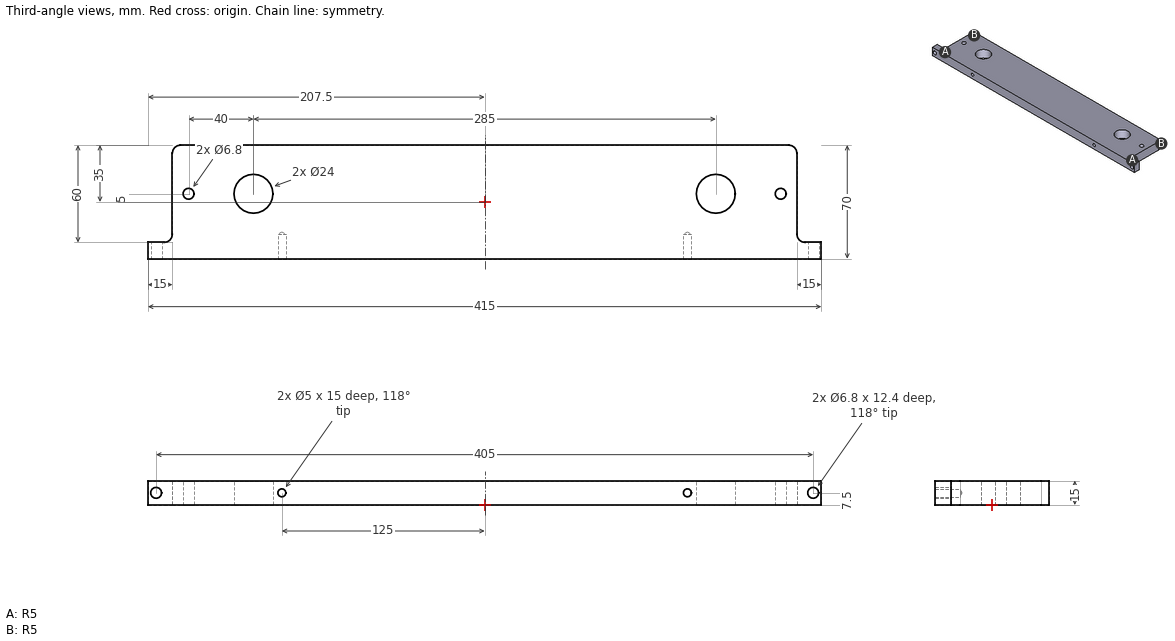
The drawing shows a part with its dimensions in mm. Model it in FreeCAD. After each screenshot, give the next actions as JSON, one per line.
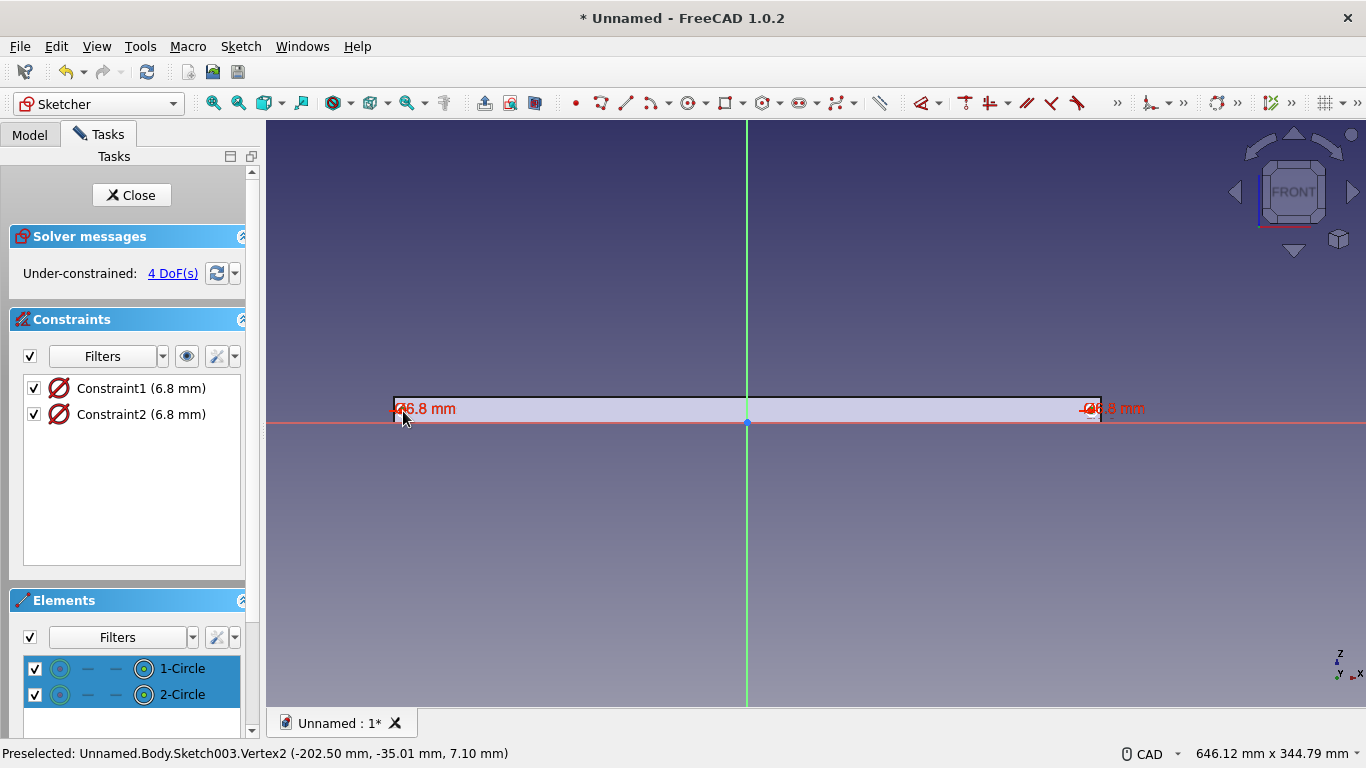
{"action": "left_click", "coordinate": [747, 641]}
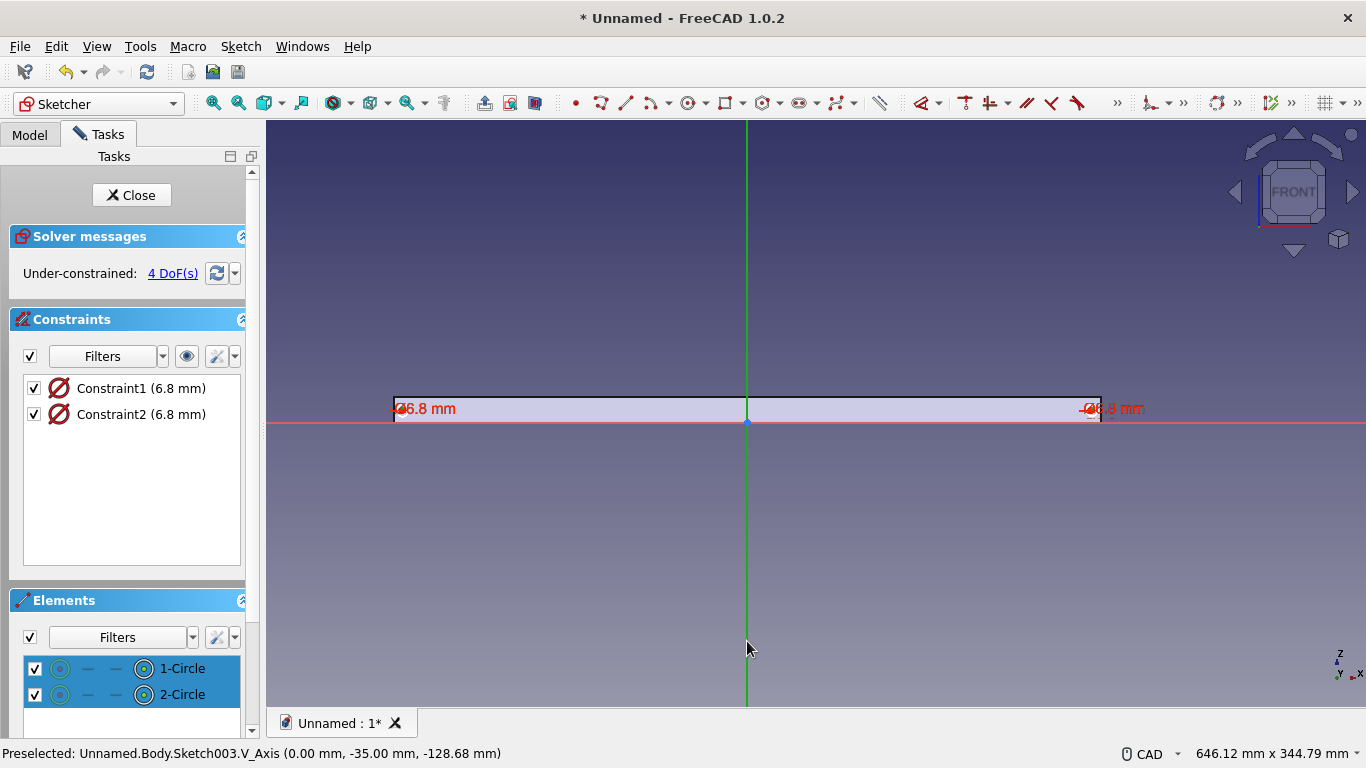
{"action": "key", "text": "s"}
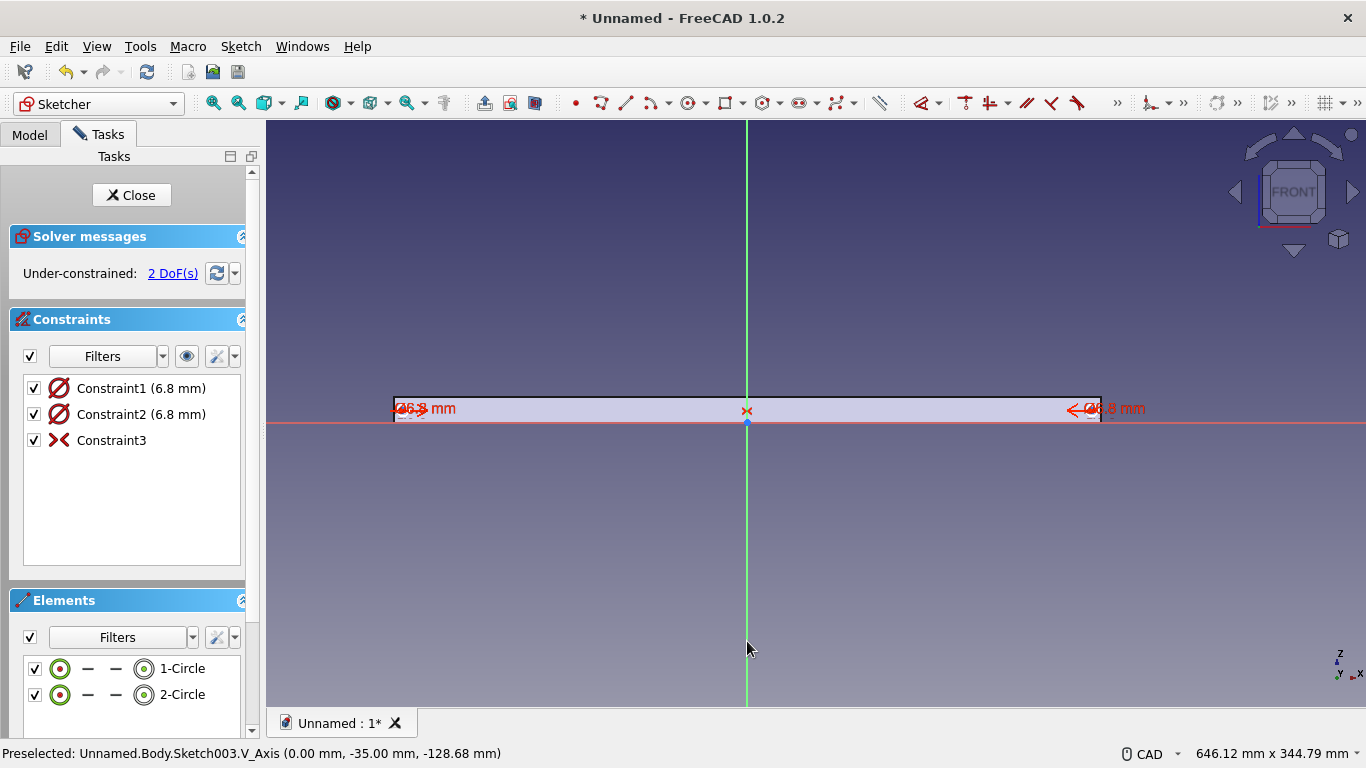
{"action": "key", "text": "d"}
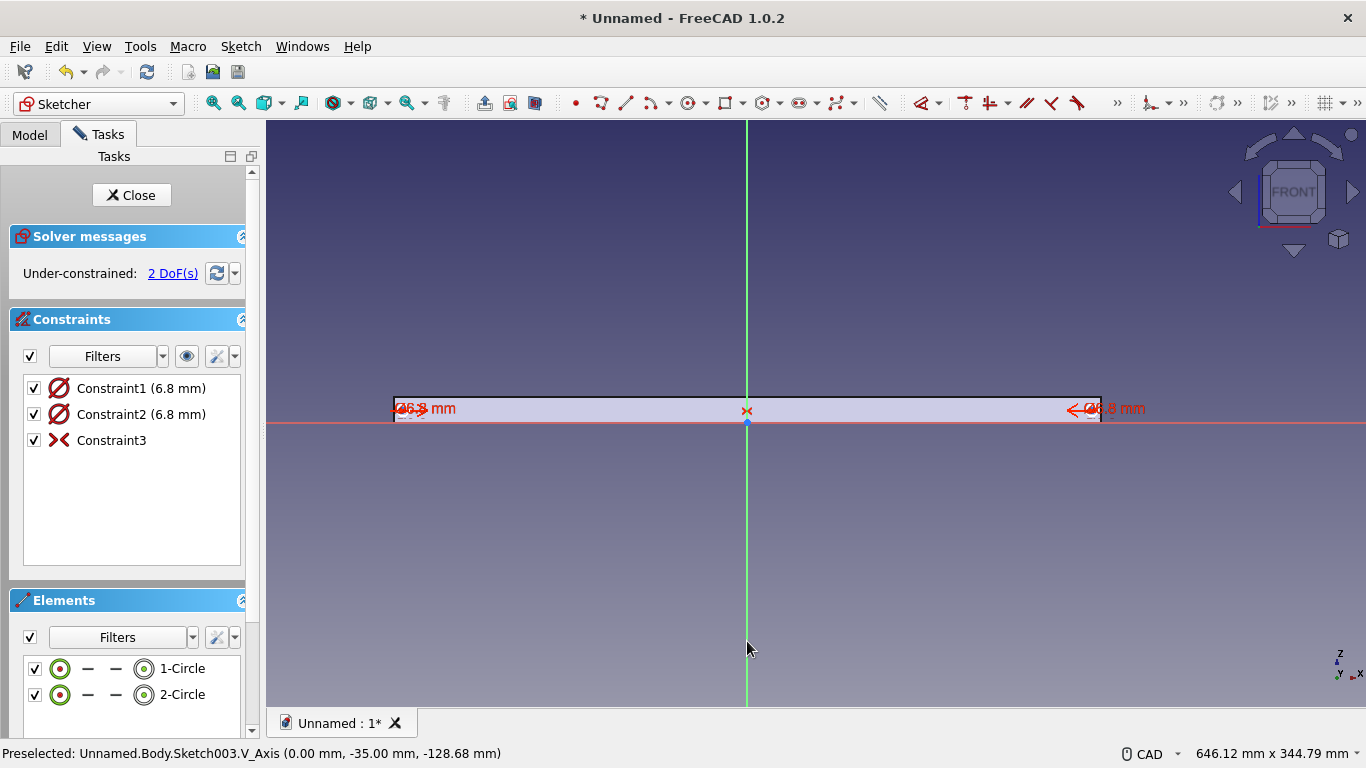
{"action": "scroll", "coordinate": [1092, 411], "scroll_direction": "up", "scroll_amount": 6}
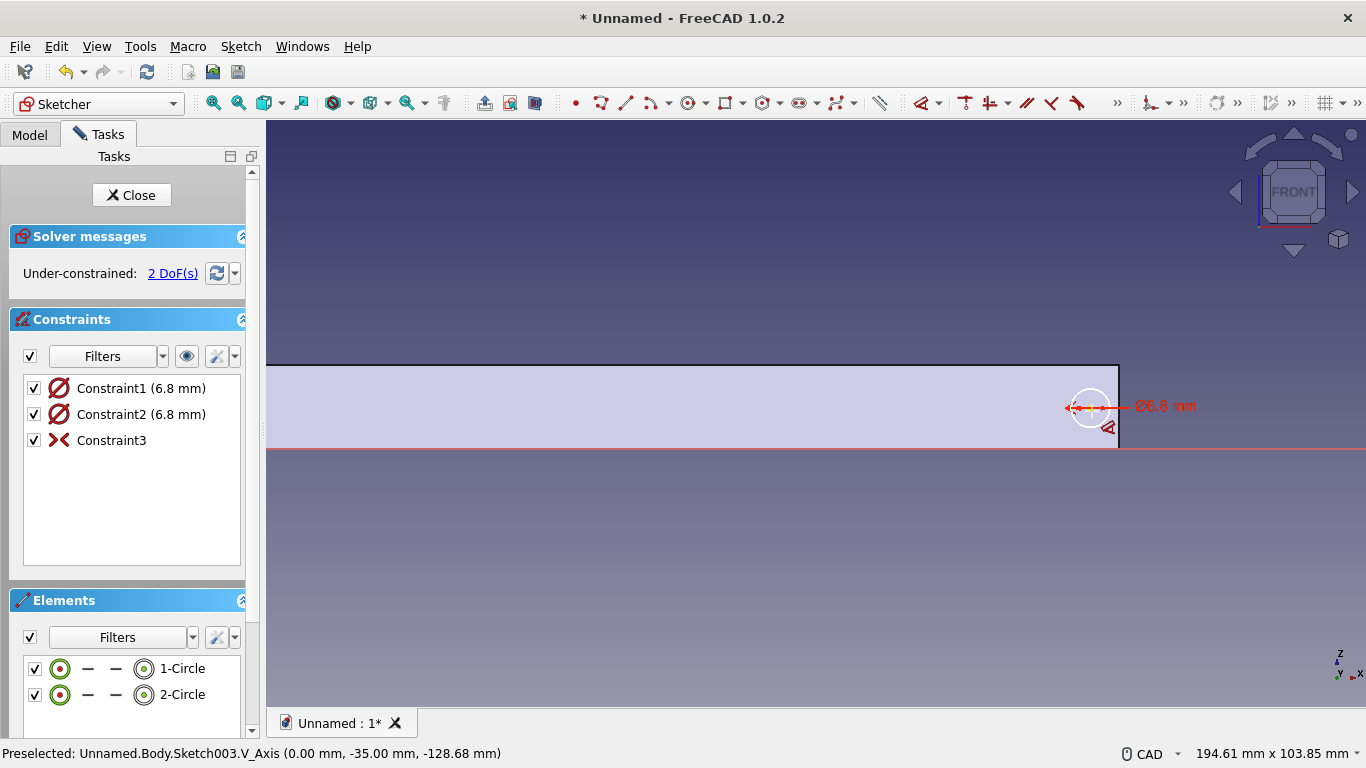
{"action": "left_click", "coordinate": [1091, 408]}
{"action": "left_click", "coordinate": [1125, 429]}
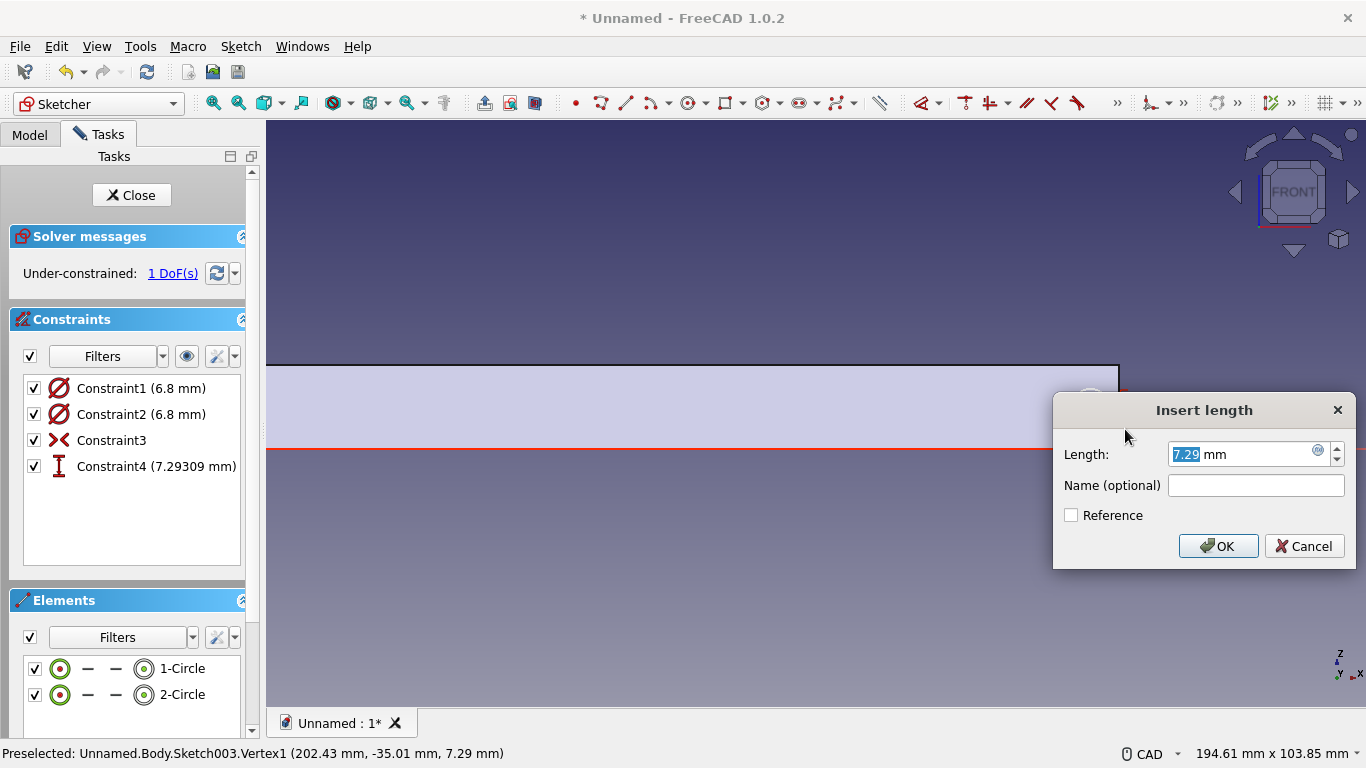
{"action": "type", "text": "7.5"}
{"action": "key", "text": "Return"}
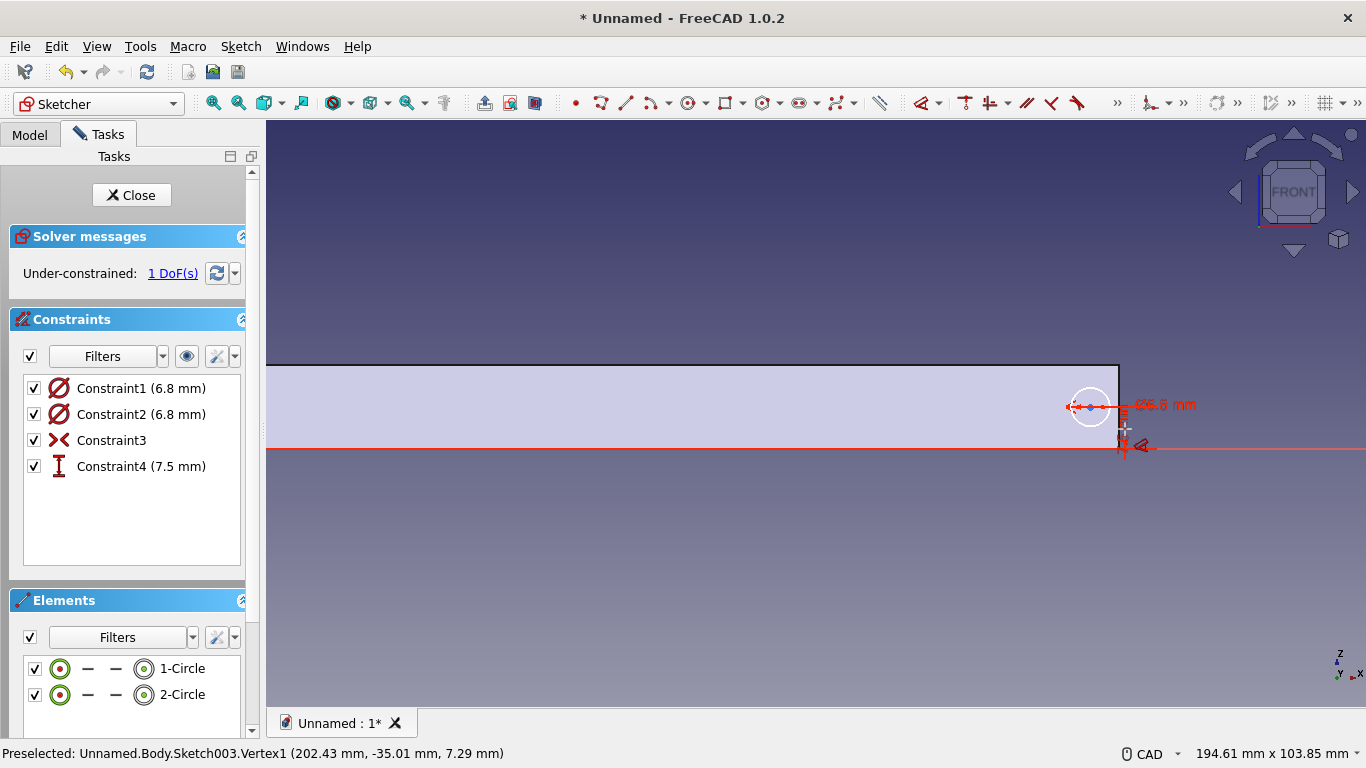
{"action": "scroll", "coordinate": [1093, 411], "scroll_direction": "down", "scroll_amount": 6}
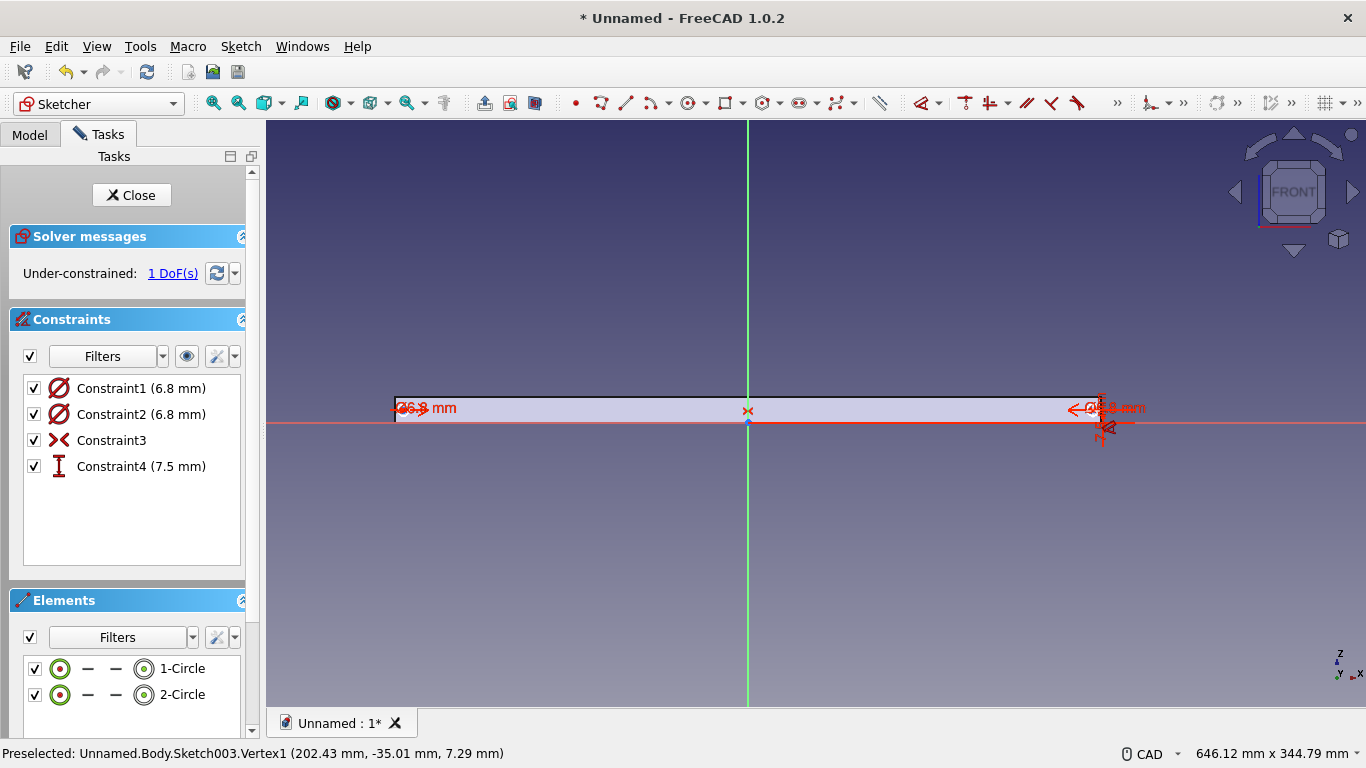
{"action": "left_click", "coordinate": [1093, 410]}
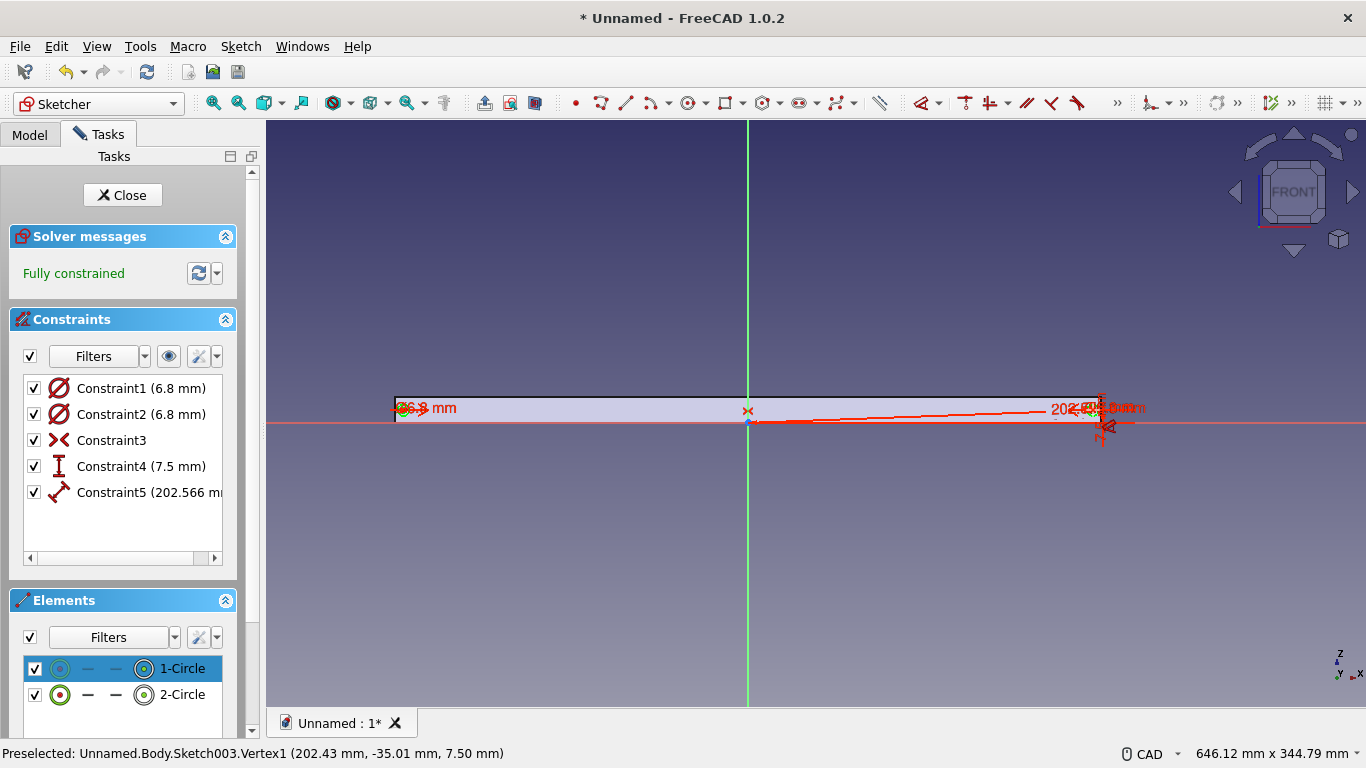
{"action": "left_click", "coordinate": [404, 410]}
{"action": "left_click", "coordinate": [590, 376]}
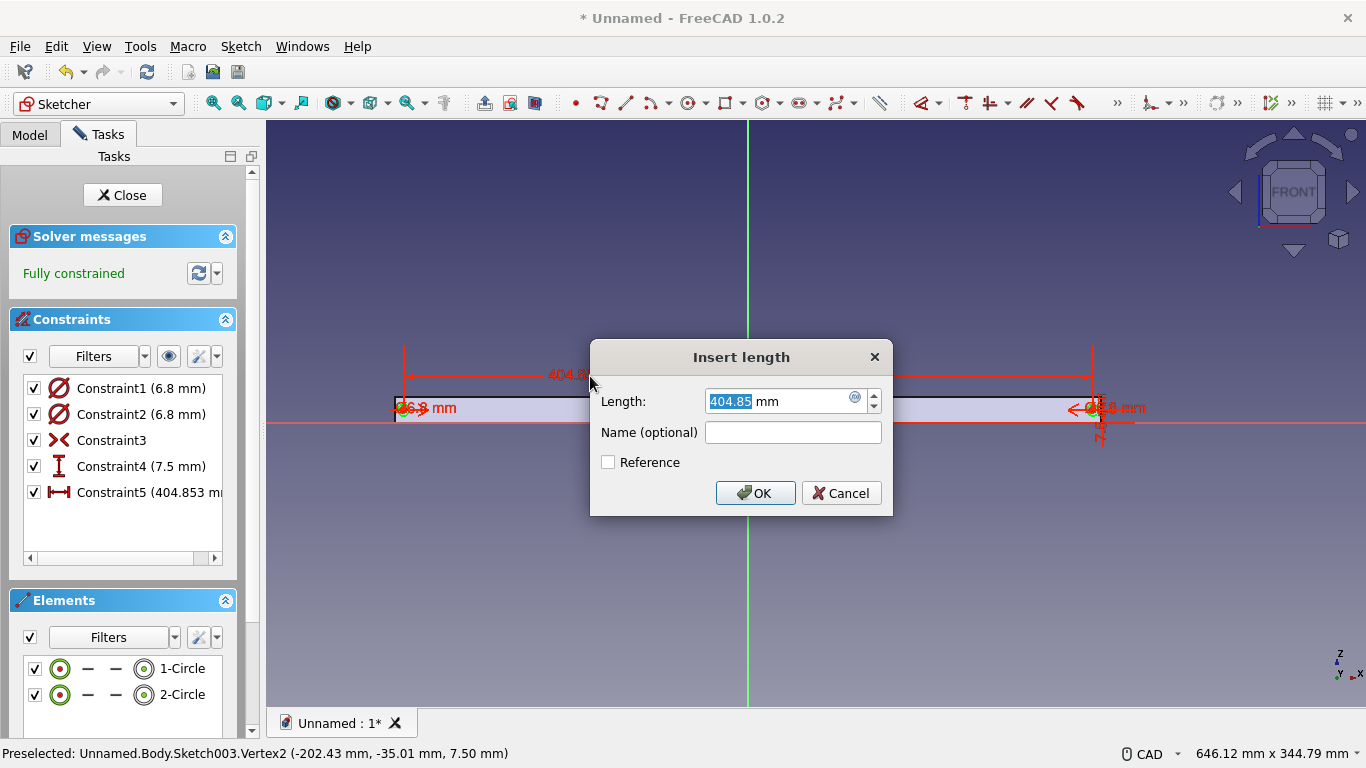
{"action": "type", "text": "405"}
{"action": "key", "text": "Return"}
{"action": "key", "text": "Escape"}